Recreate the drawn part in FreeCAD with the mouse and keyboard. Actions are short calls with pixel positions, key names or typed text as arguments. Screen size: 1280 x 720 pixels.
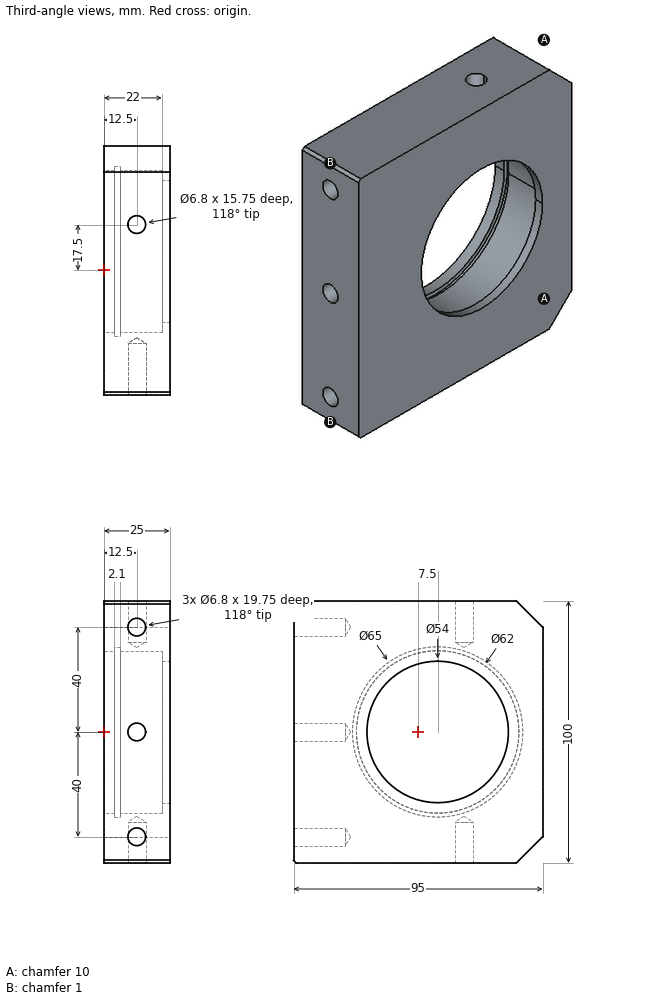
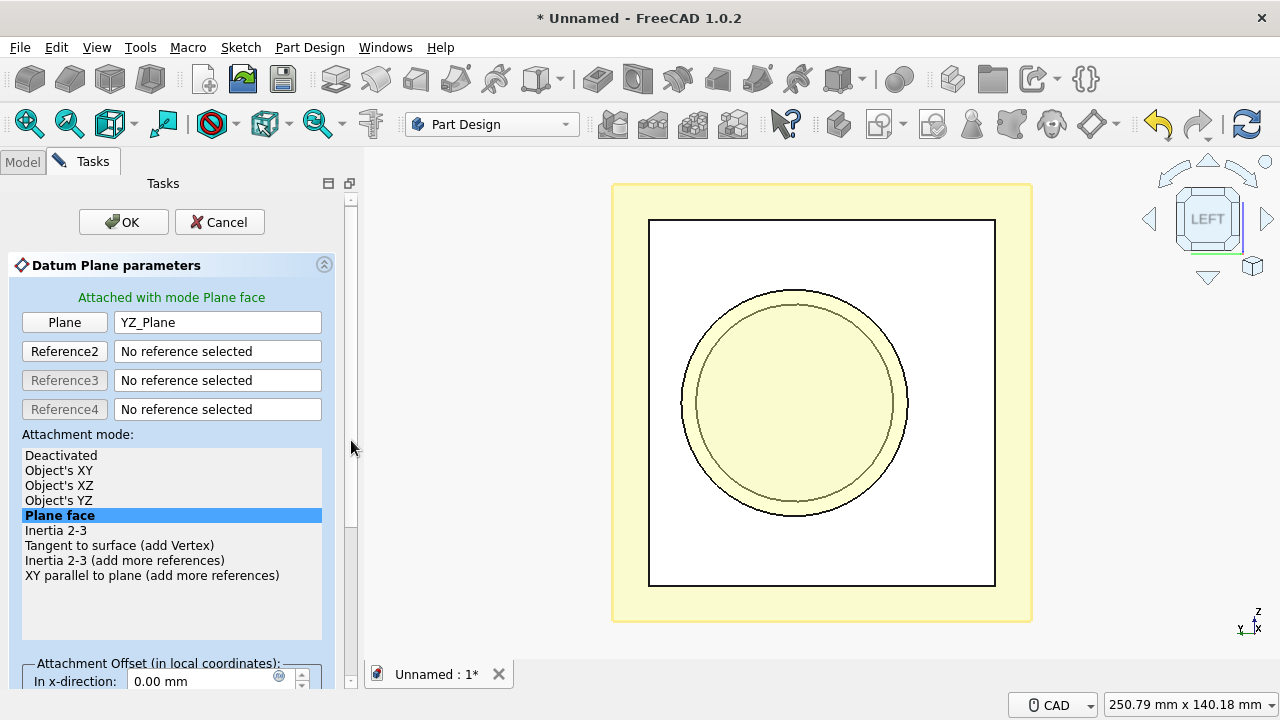
click(124, 222)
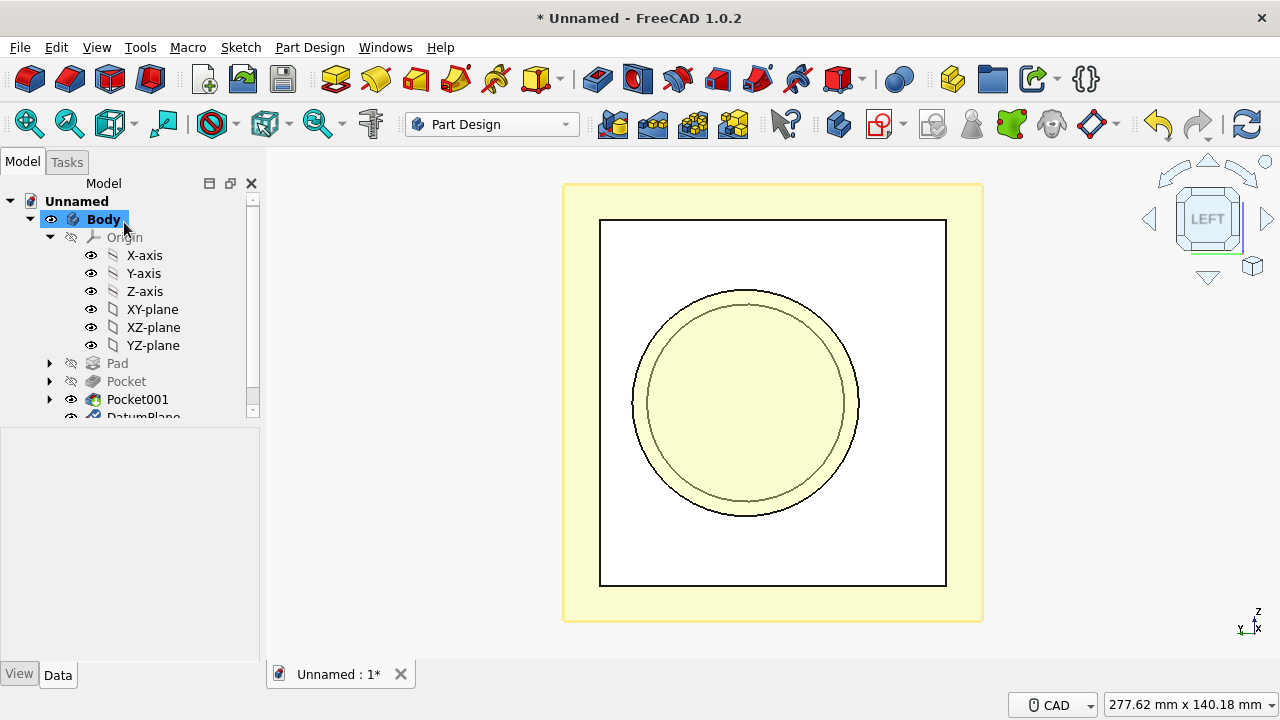
click(116, 417)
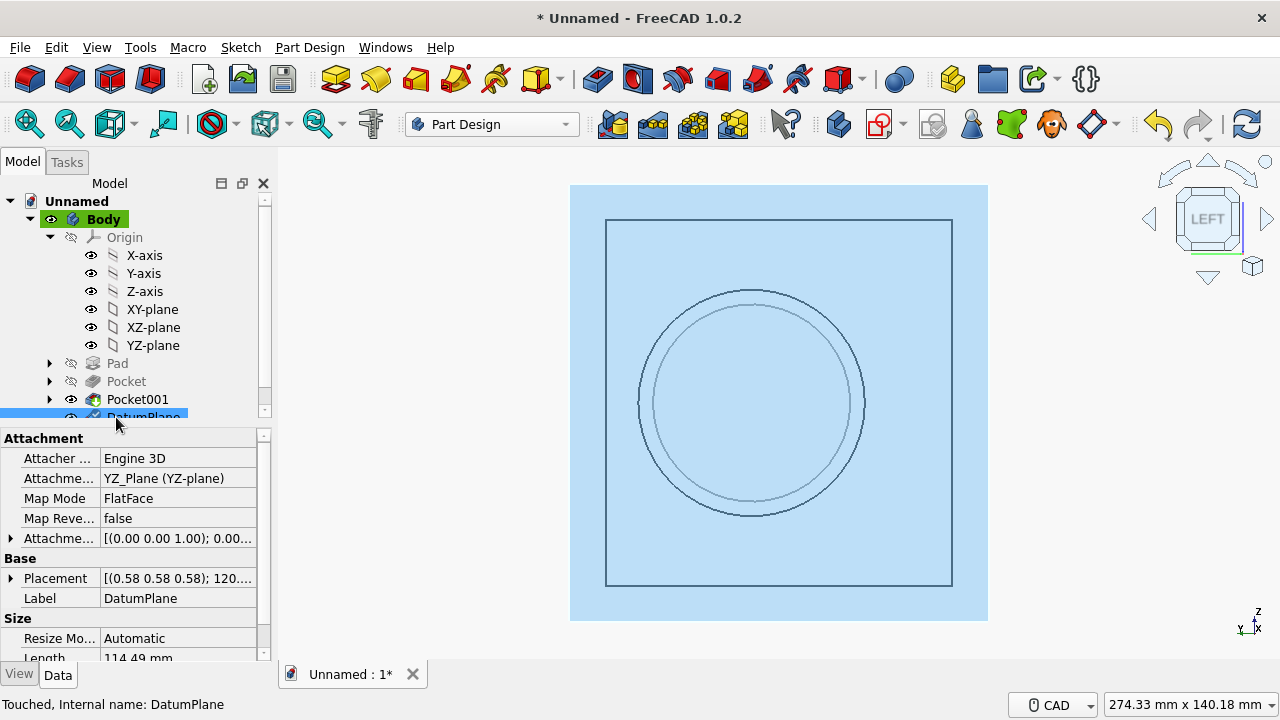
click(880, 124)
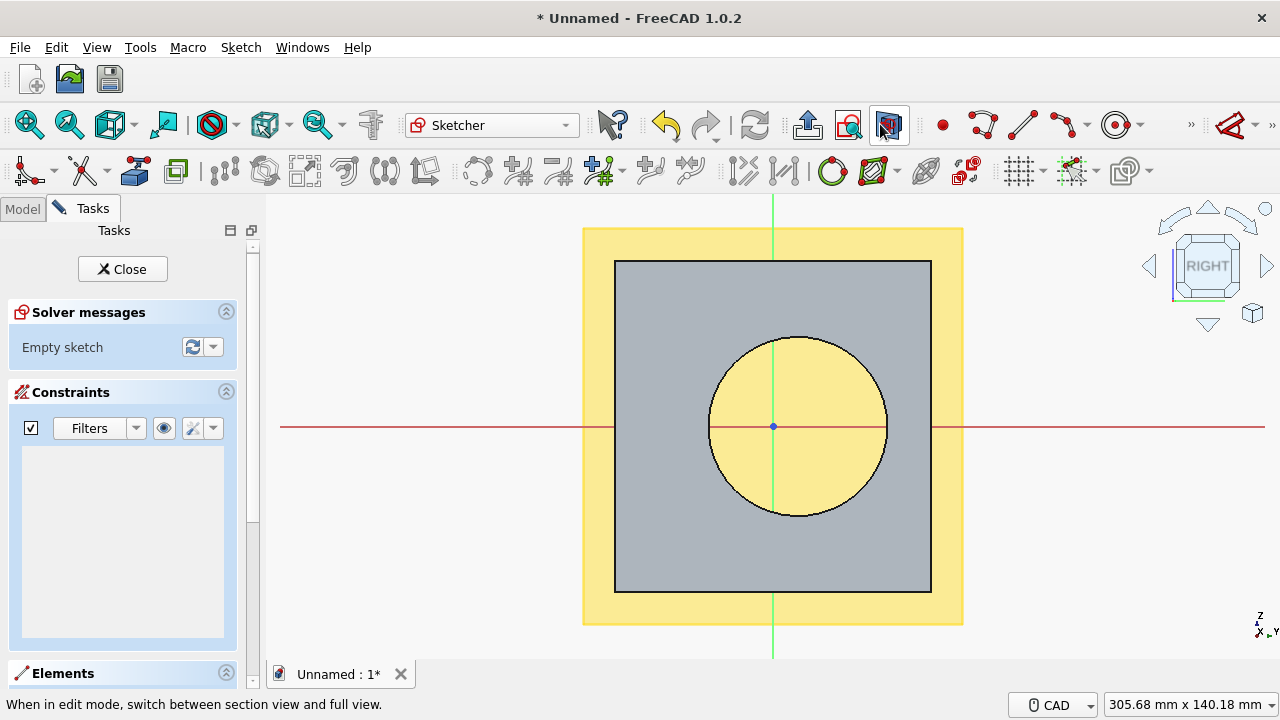
click(890, 126)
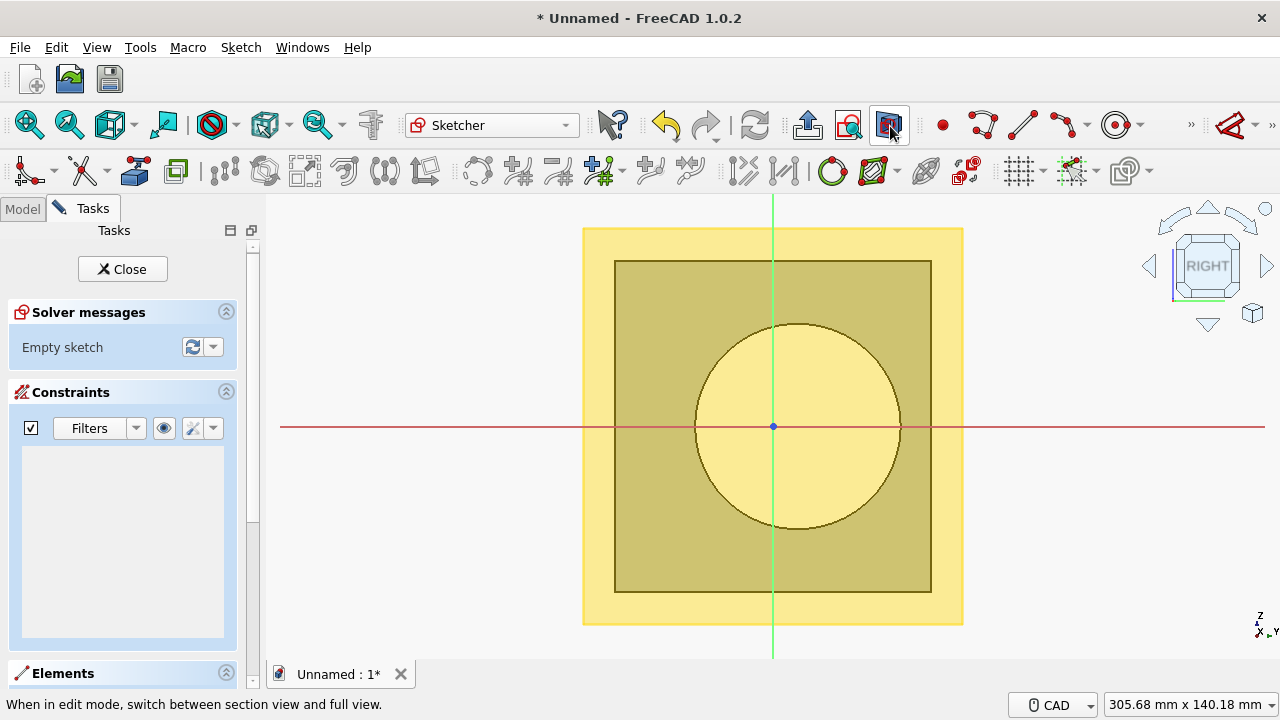
click(1116, 126)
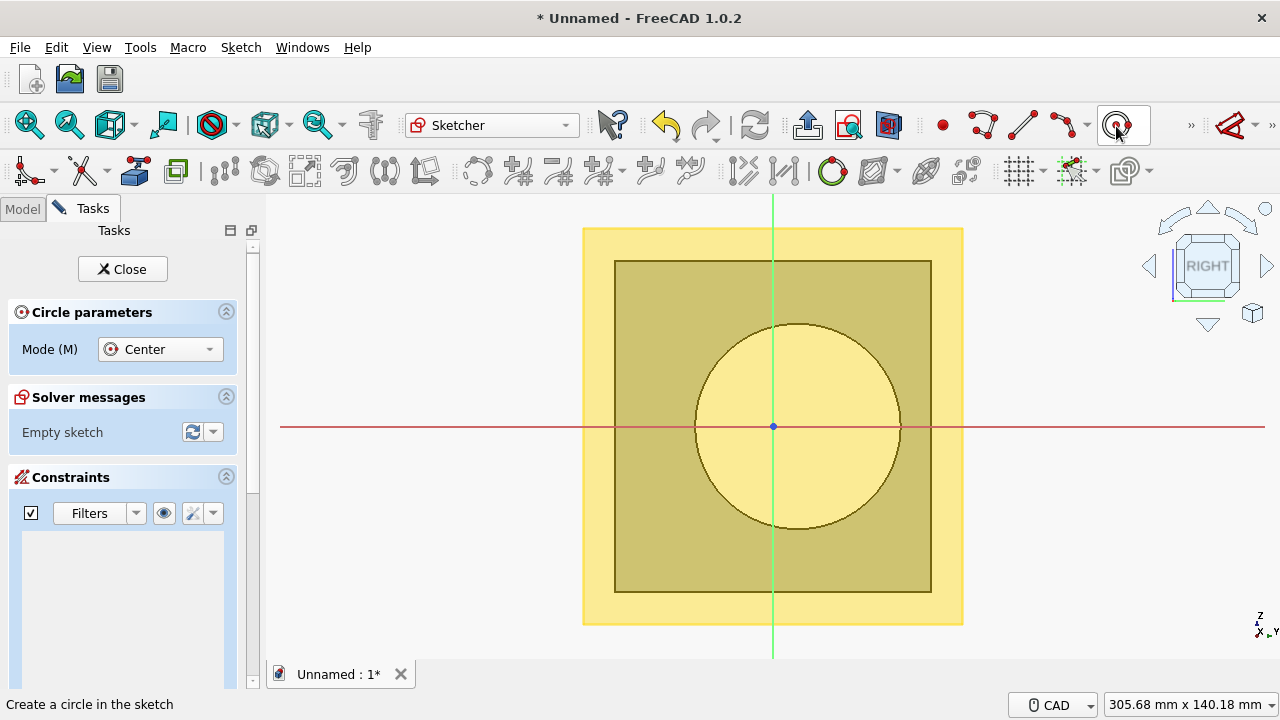
click(798, 427)
click(874, 350)
key(Escape)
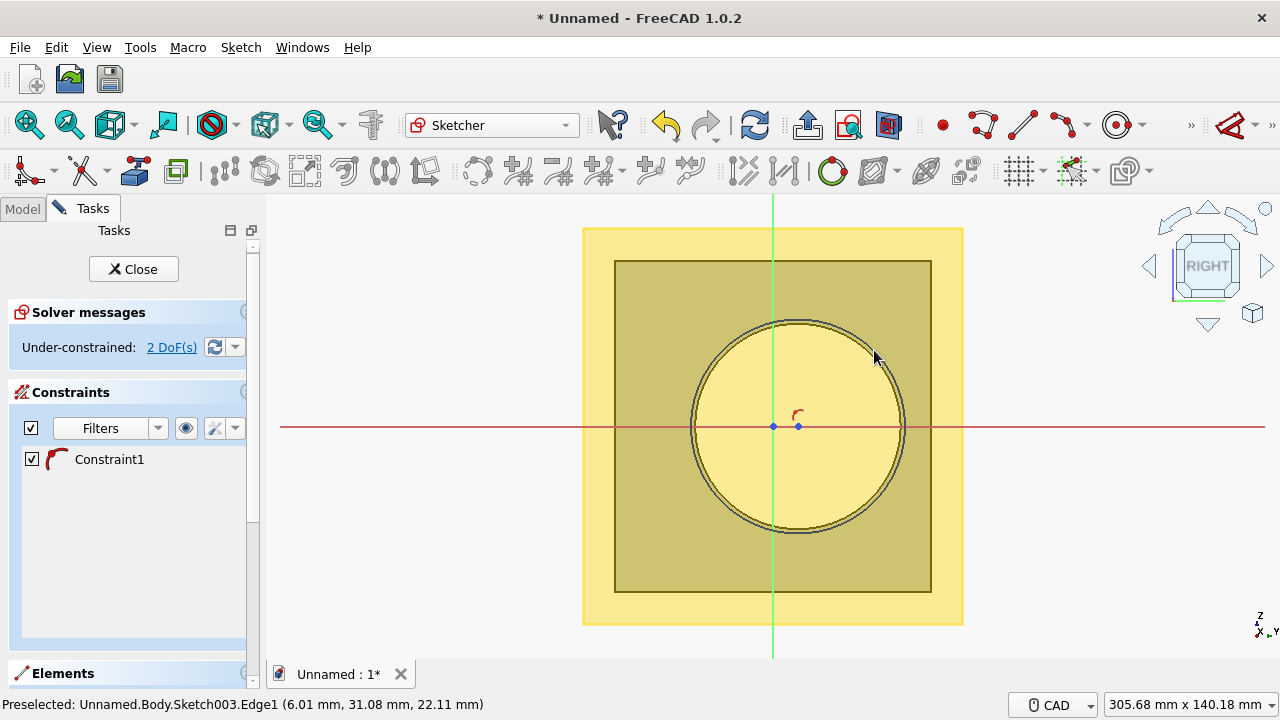
click(1230, 126)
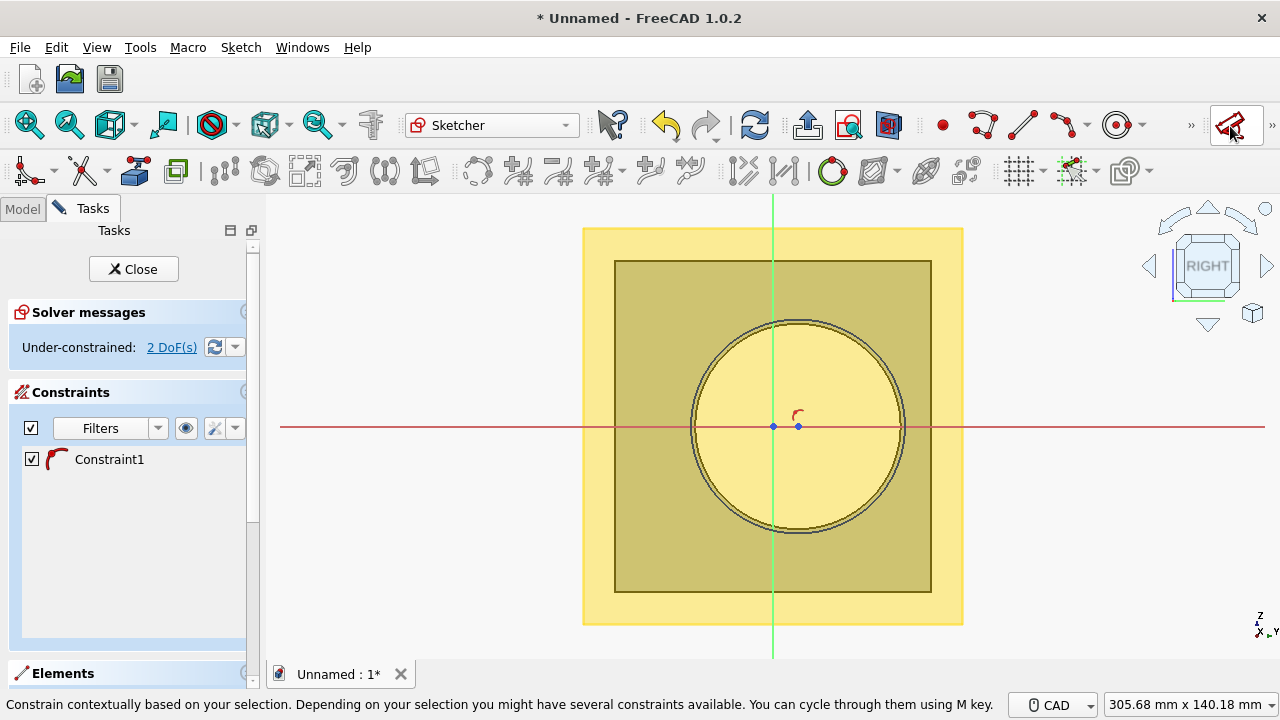
click(874, 351)
click(897, 328)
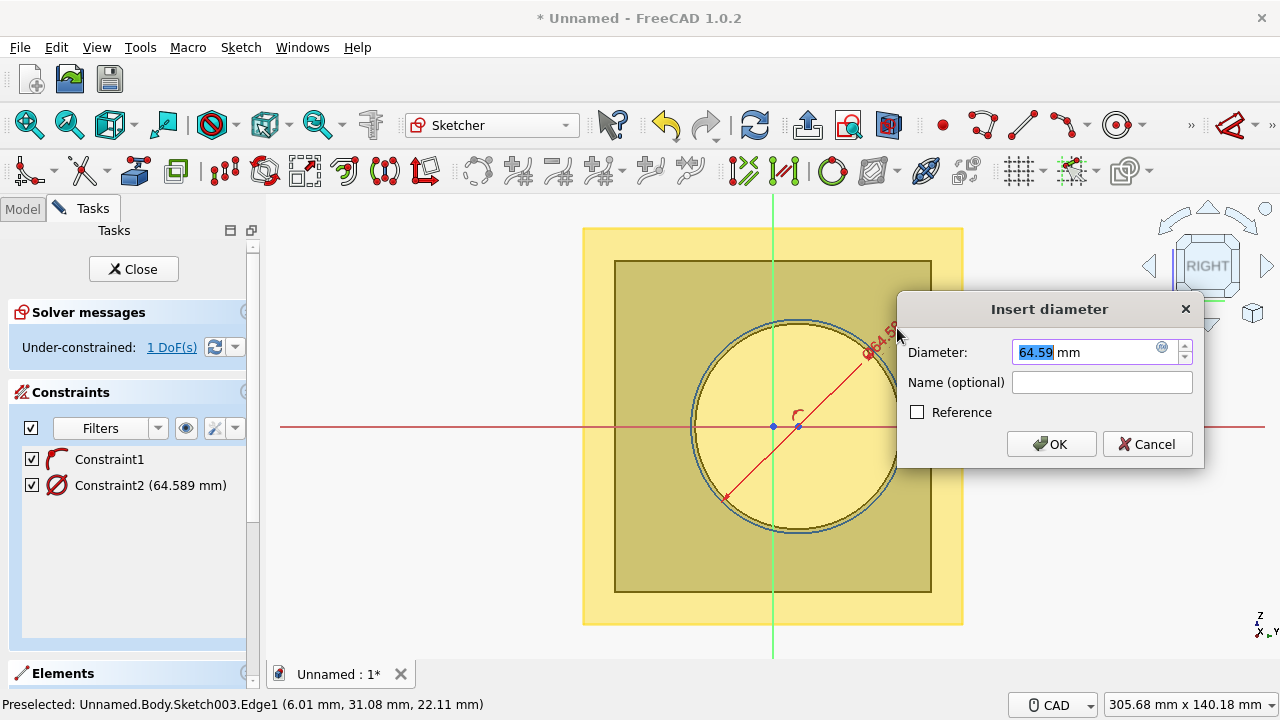
text(65)
key(Return)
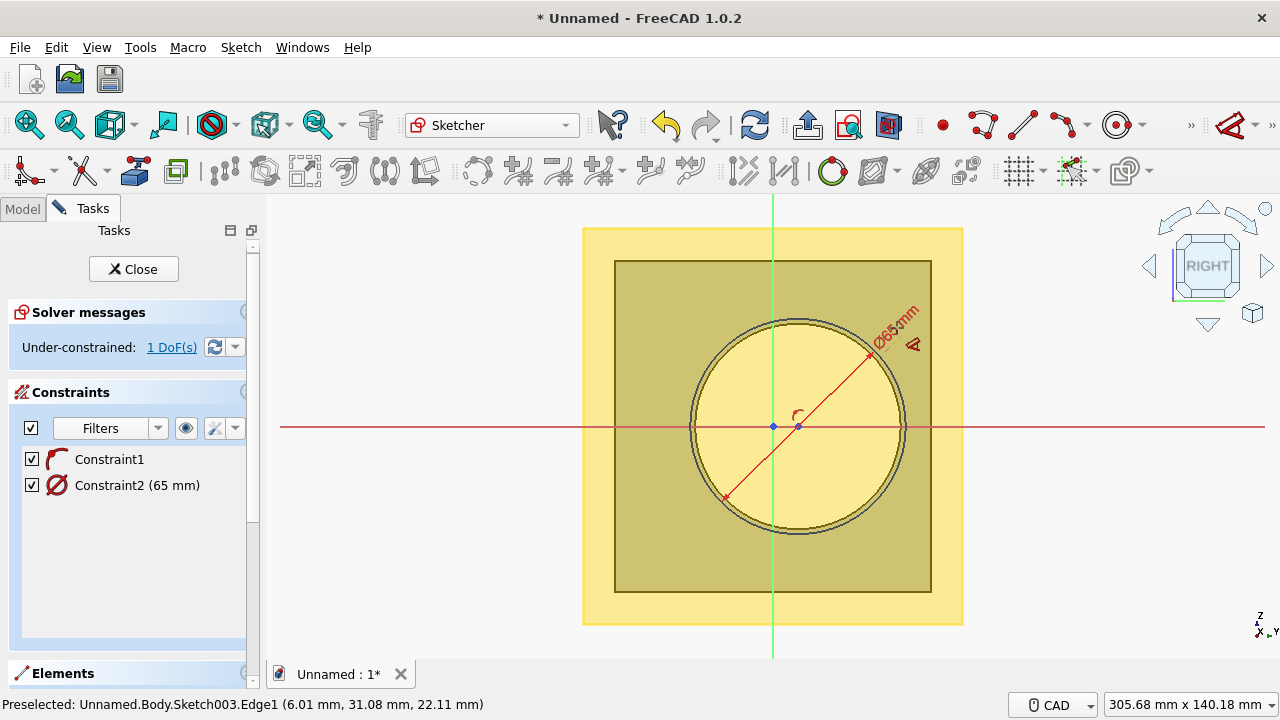
scroll(798, 427, up, 3)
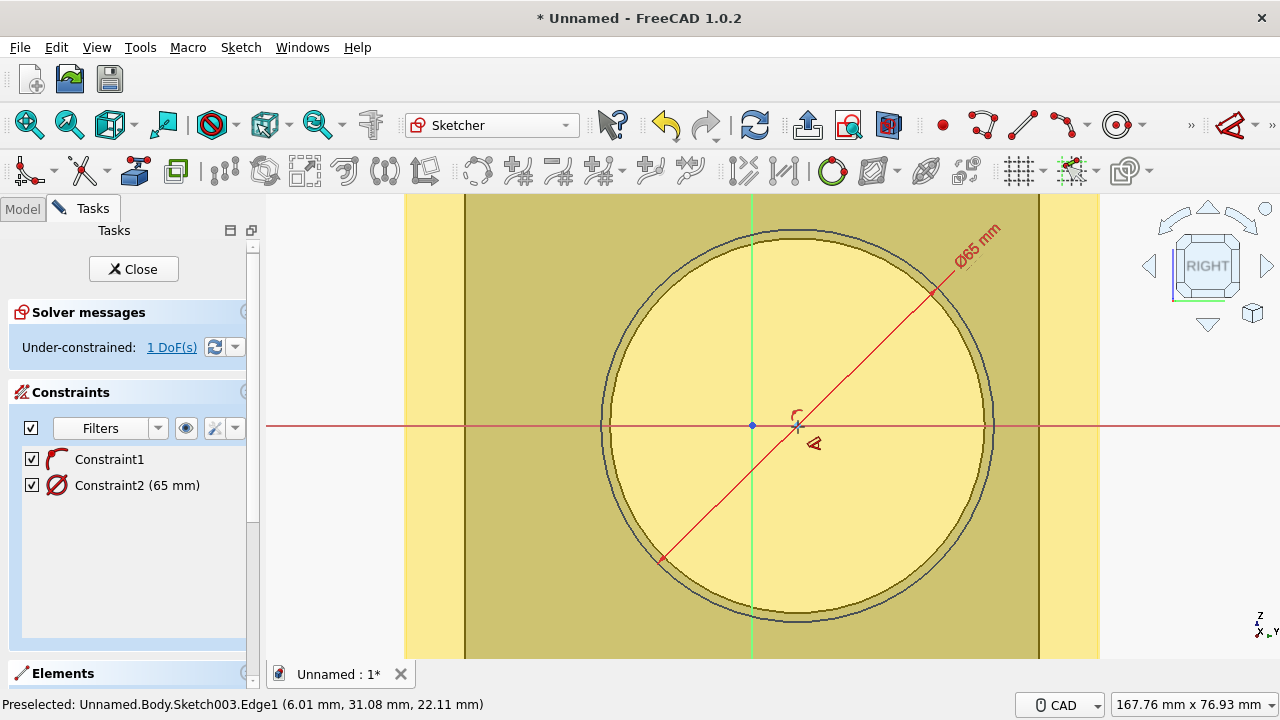
click(798, 426)
click(775, 460)